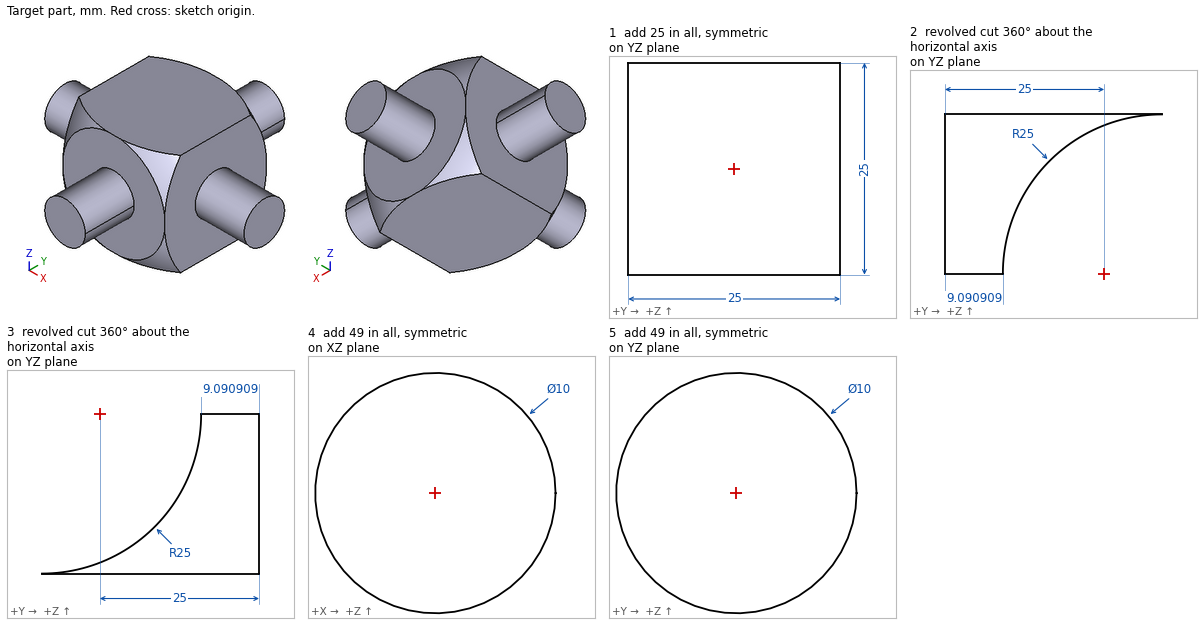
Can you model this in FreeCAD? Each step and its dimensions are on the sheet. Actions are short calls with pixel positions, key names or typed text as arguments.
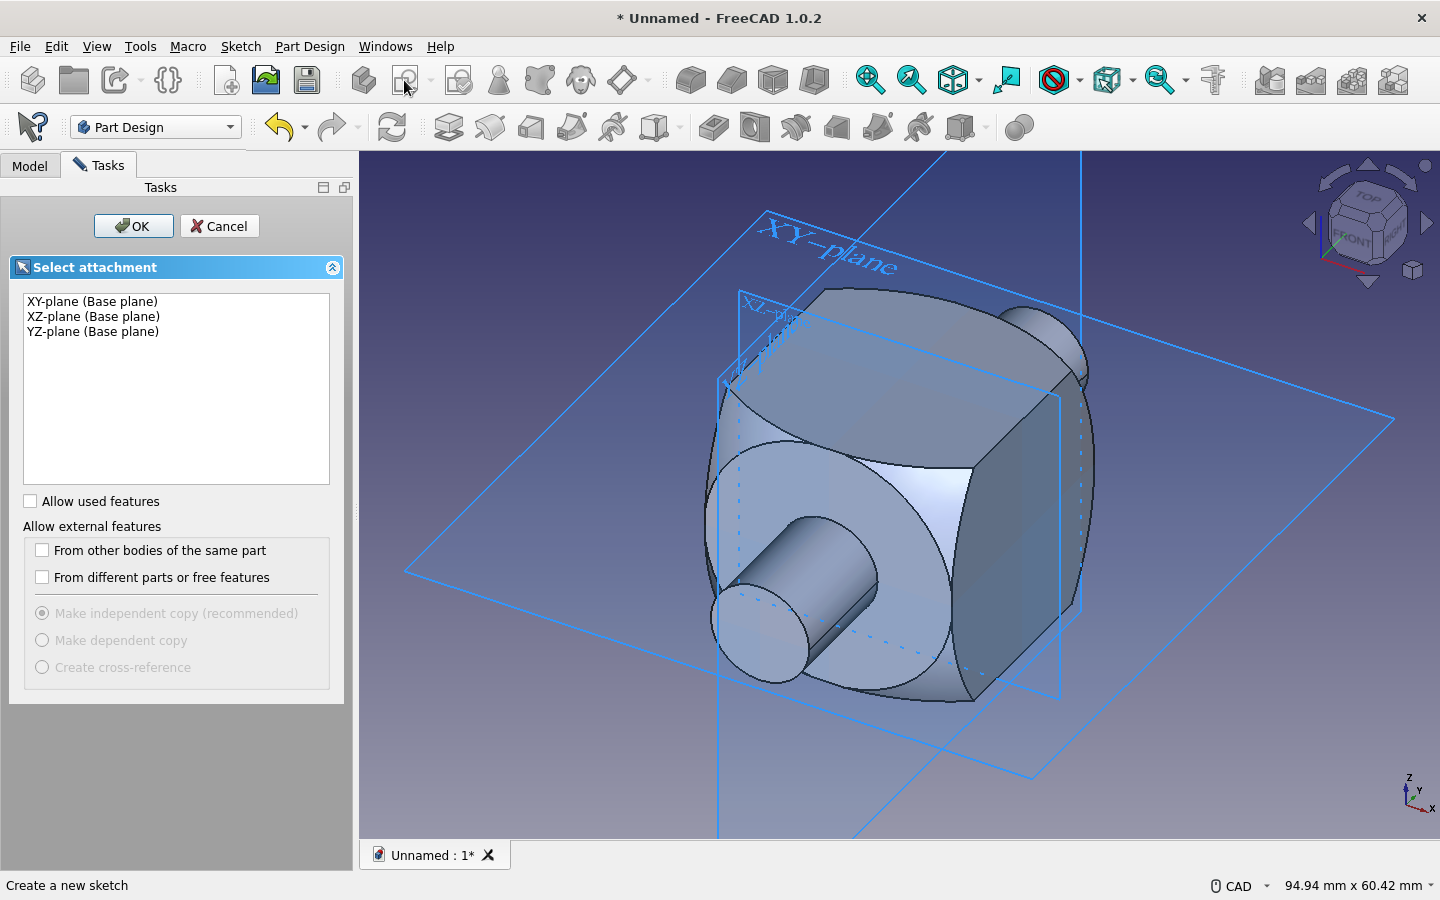
click(84, 332)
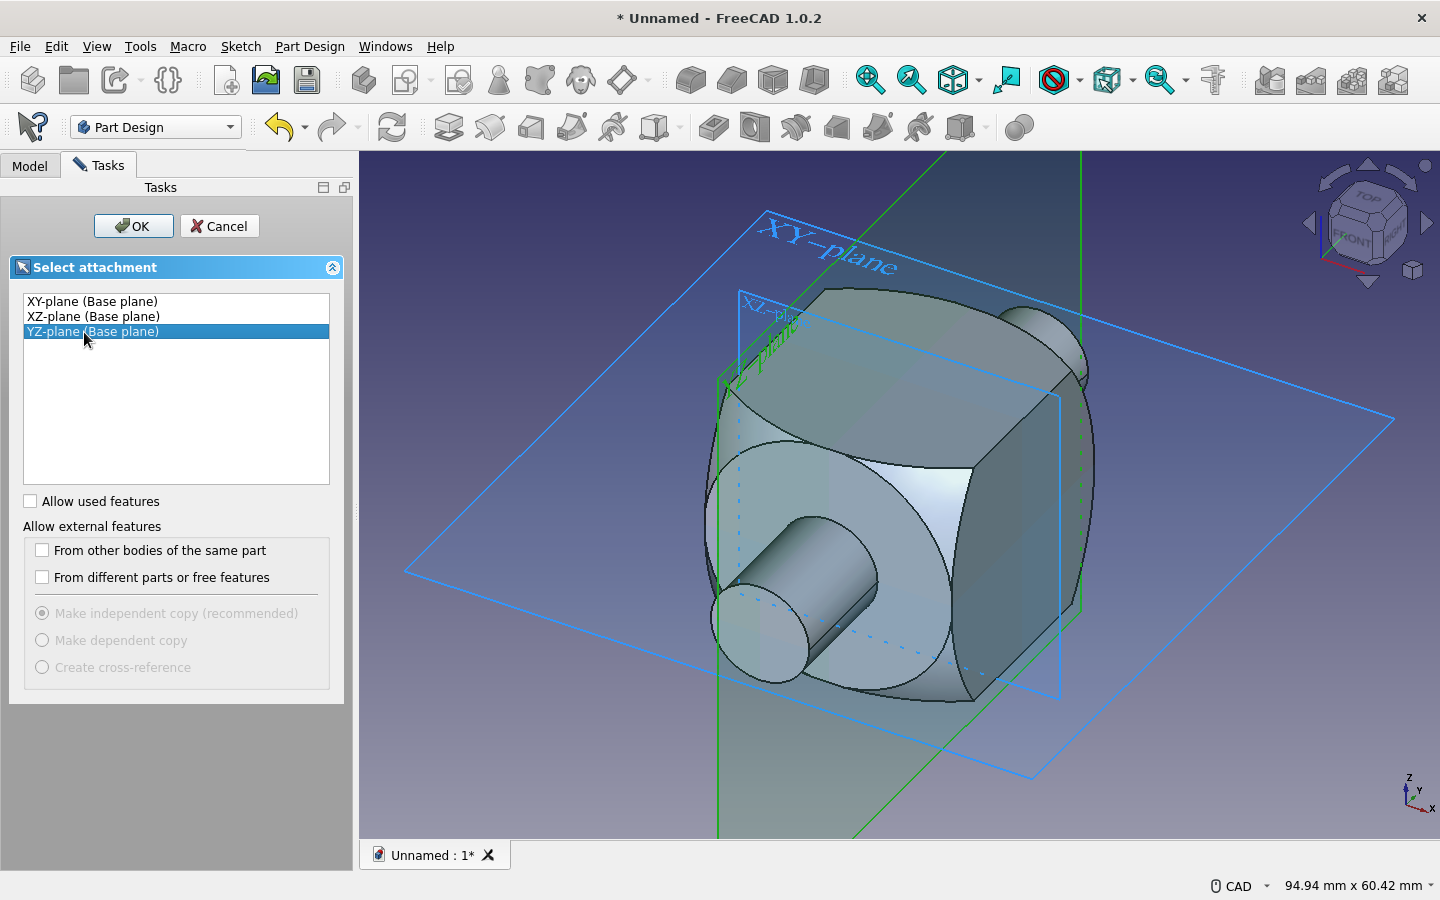
click(134, 226)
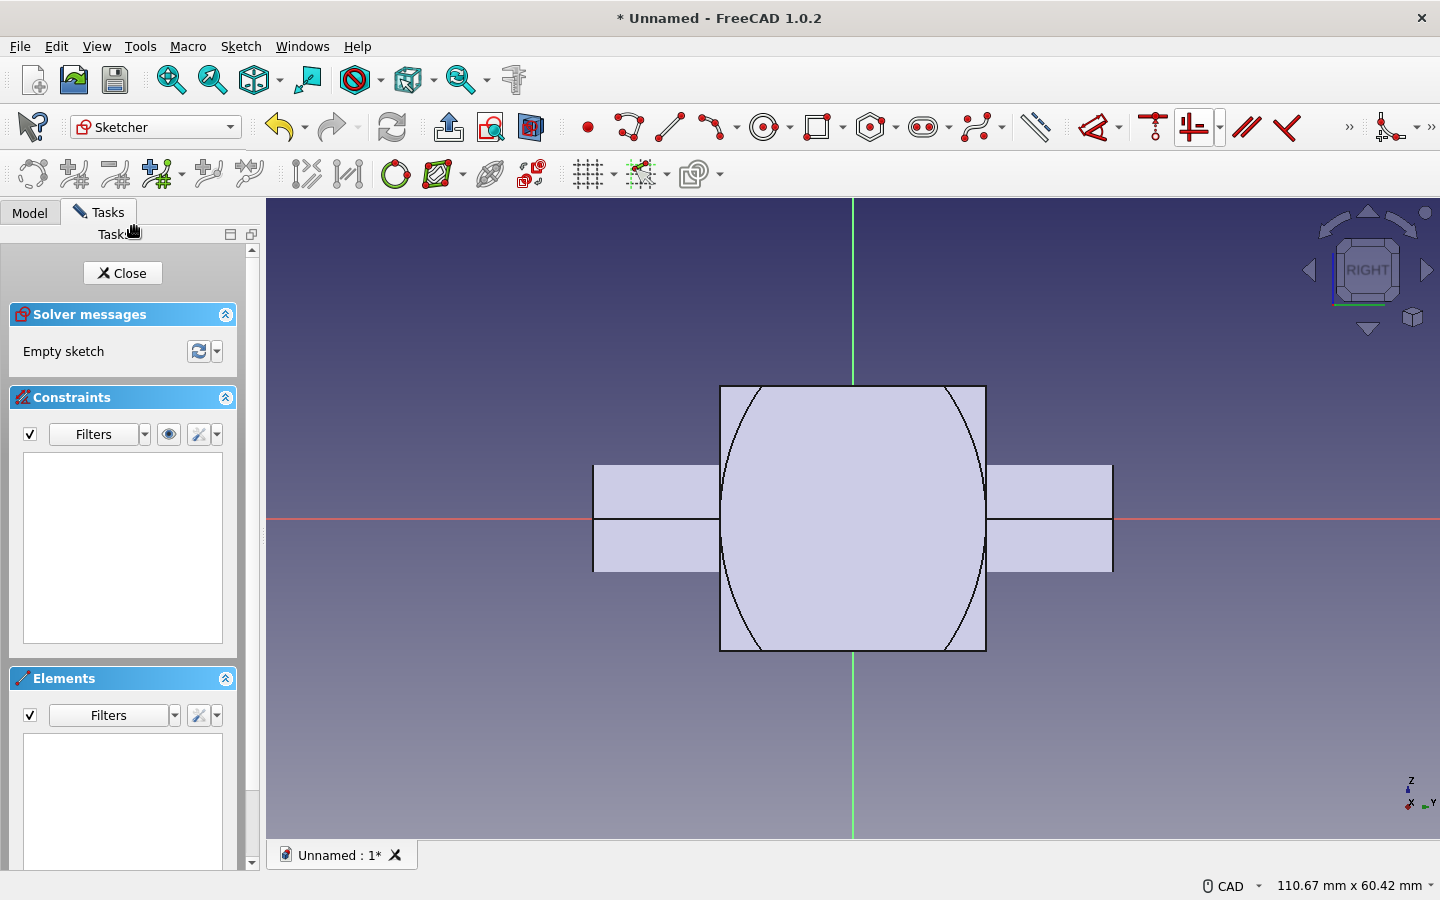
click(531, 128)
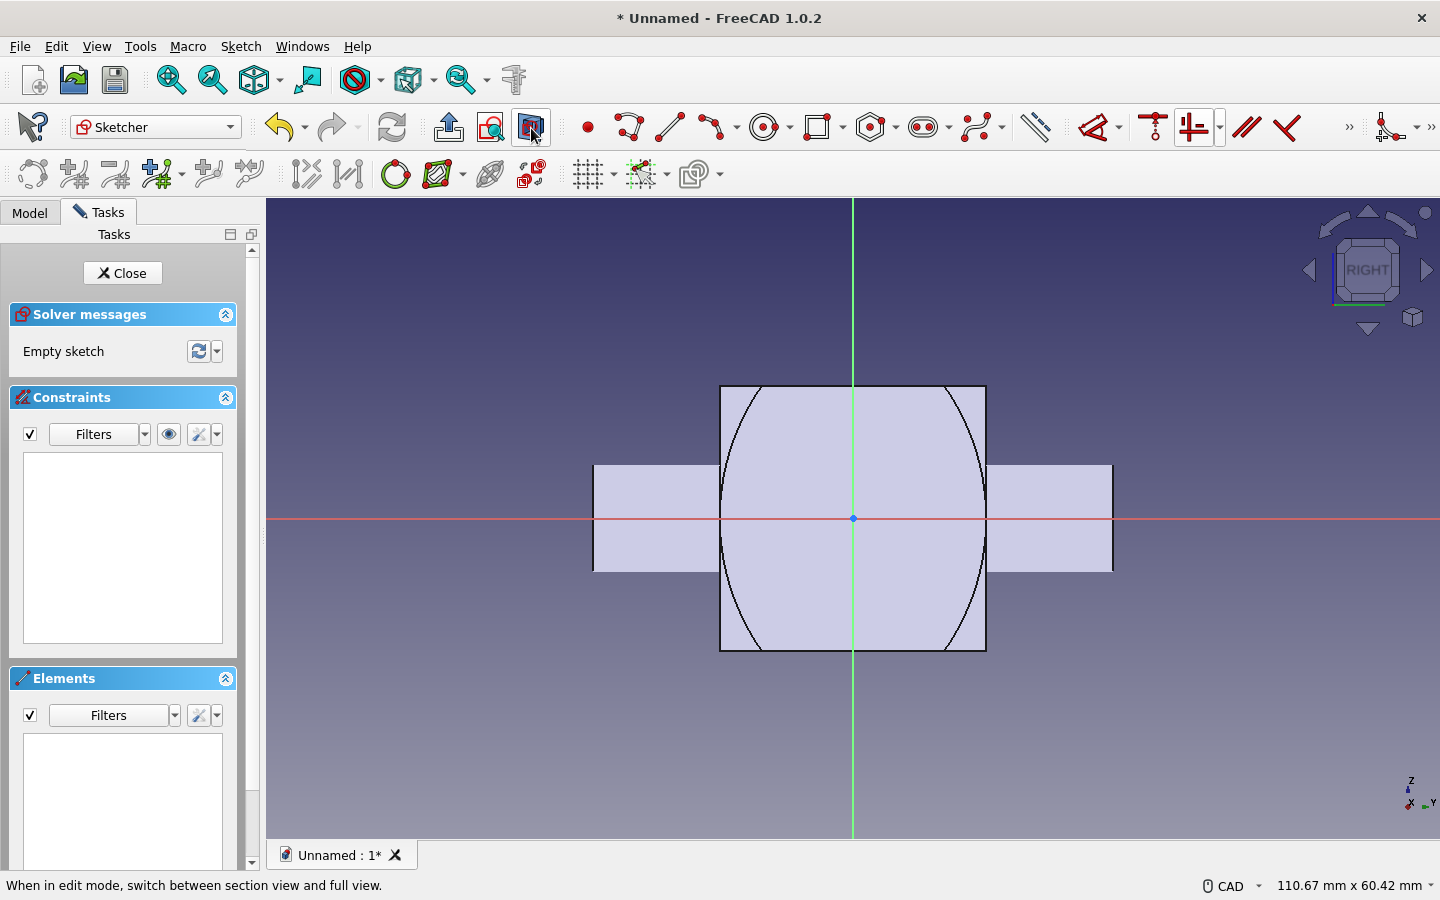
scroll(875, 518, up, 7)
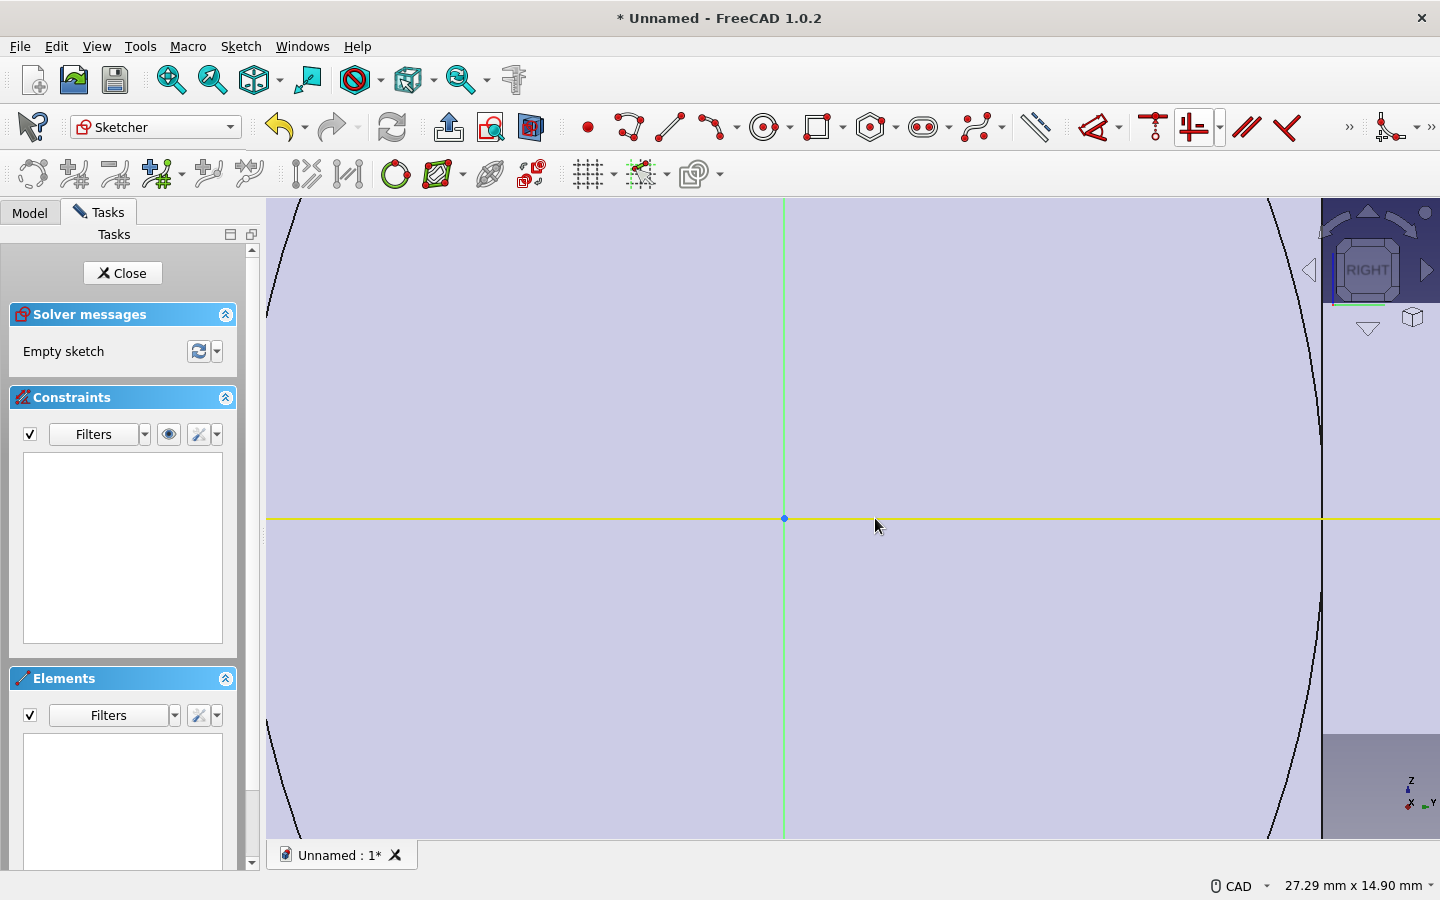
key(g)
key(c)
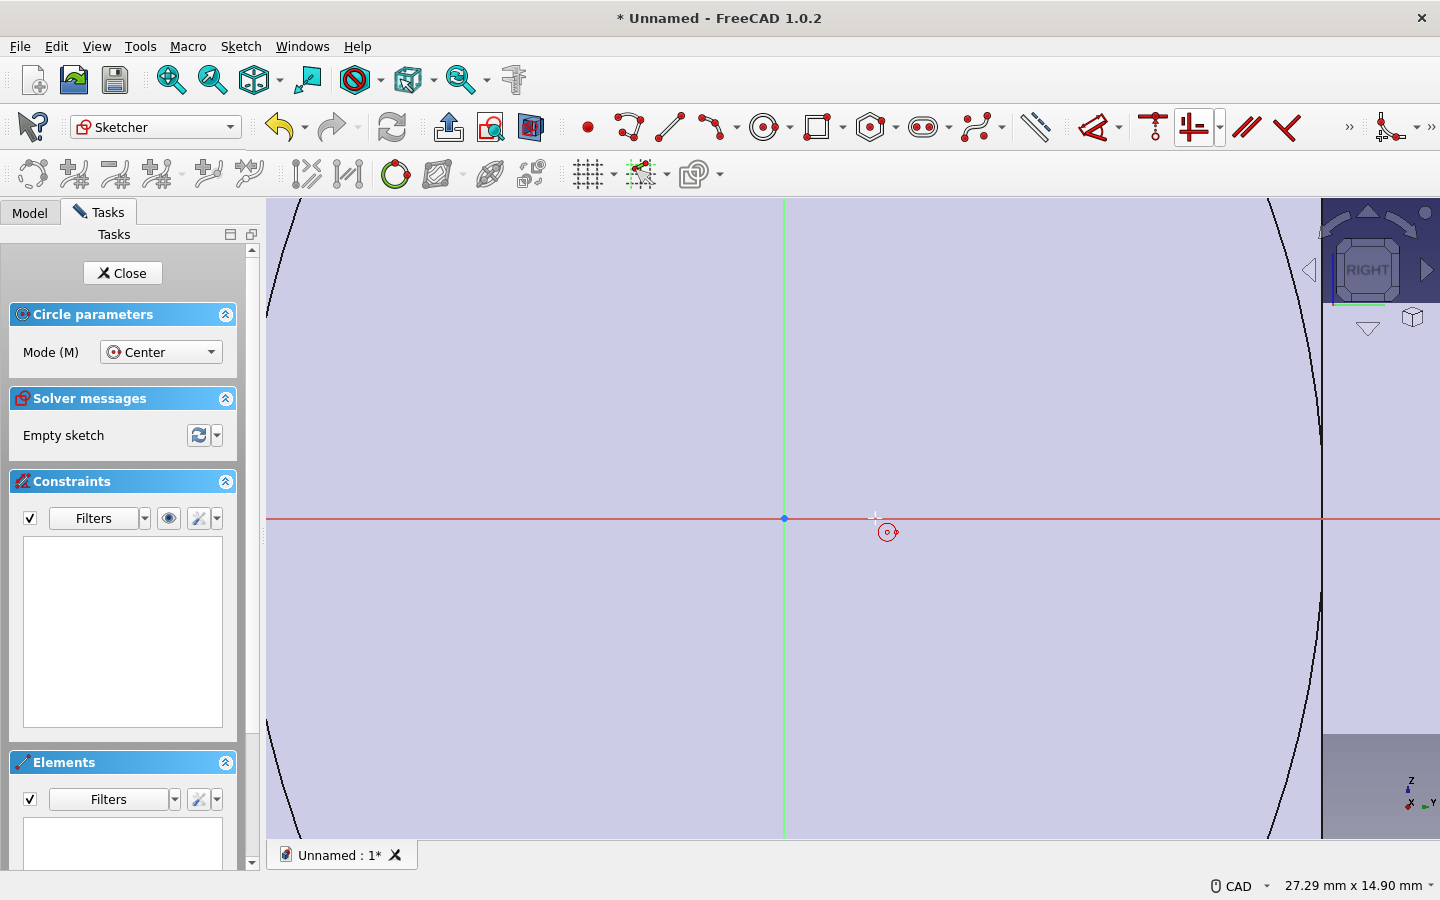
click(784, 518)
click(936, 366)
key(Escape)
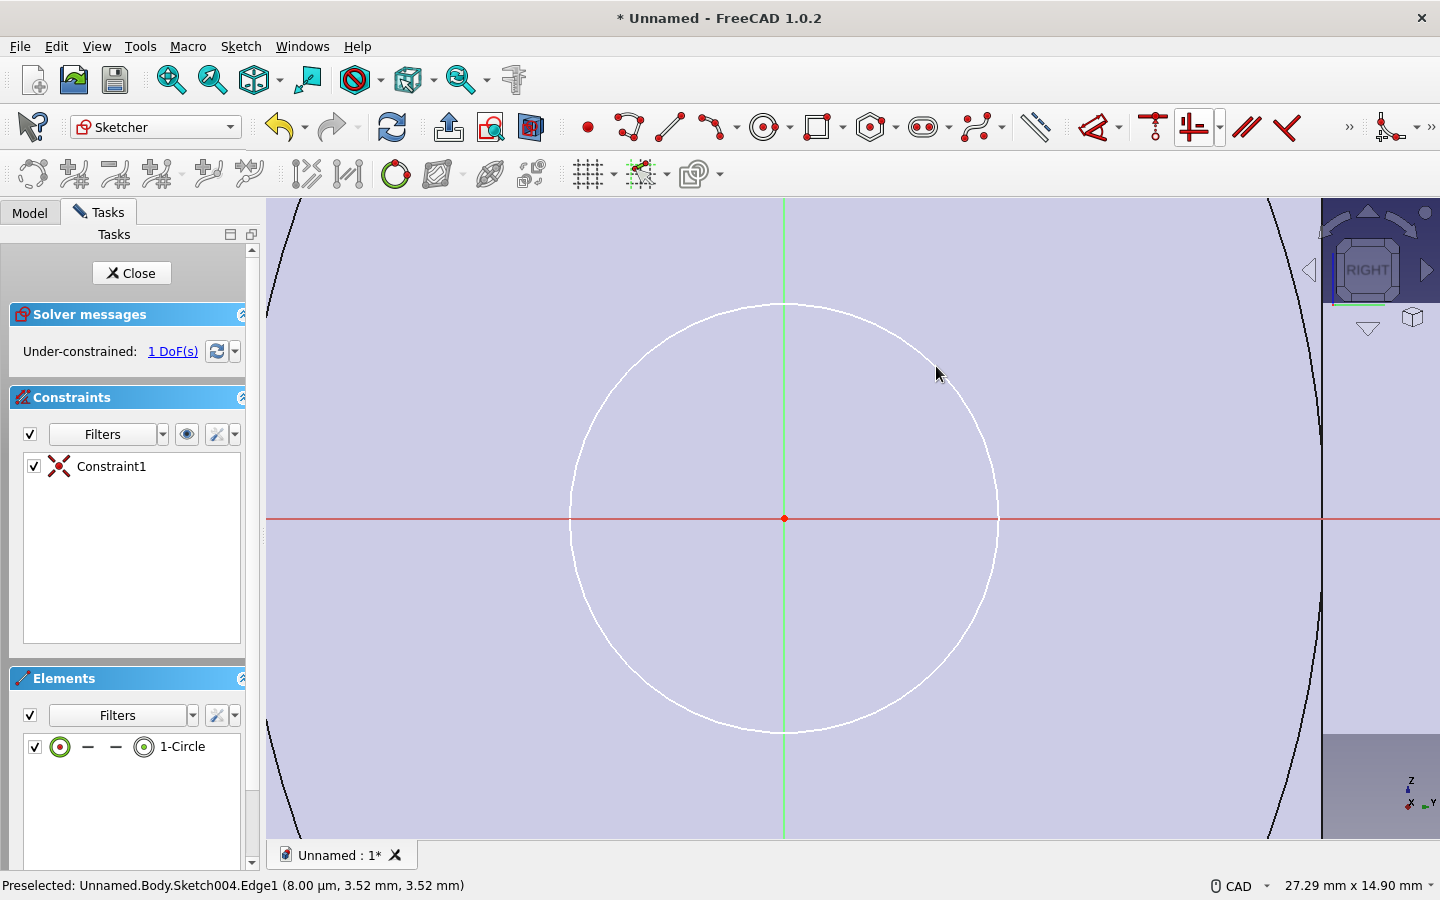
click(1092, 128)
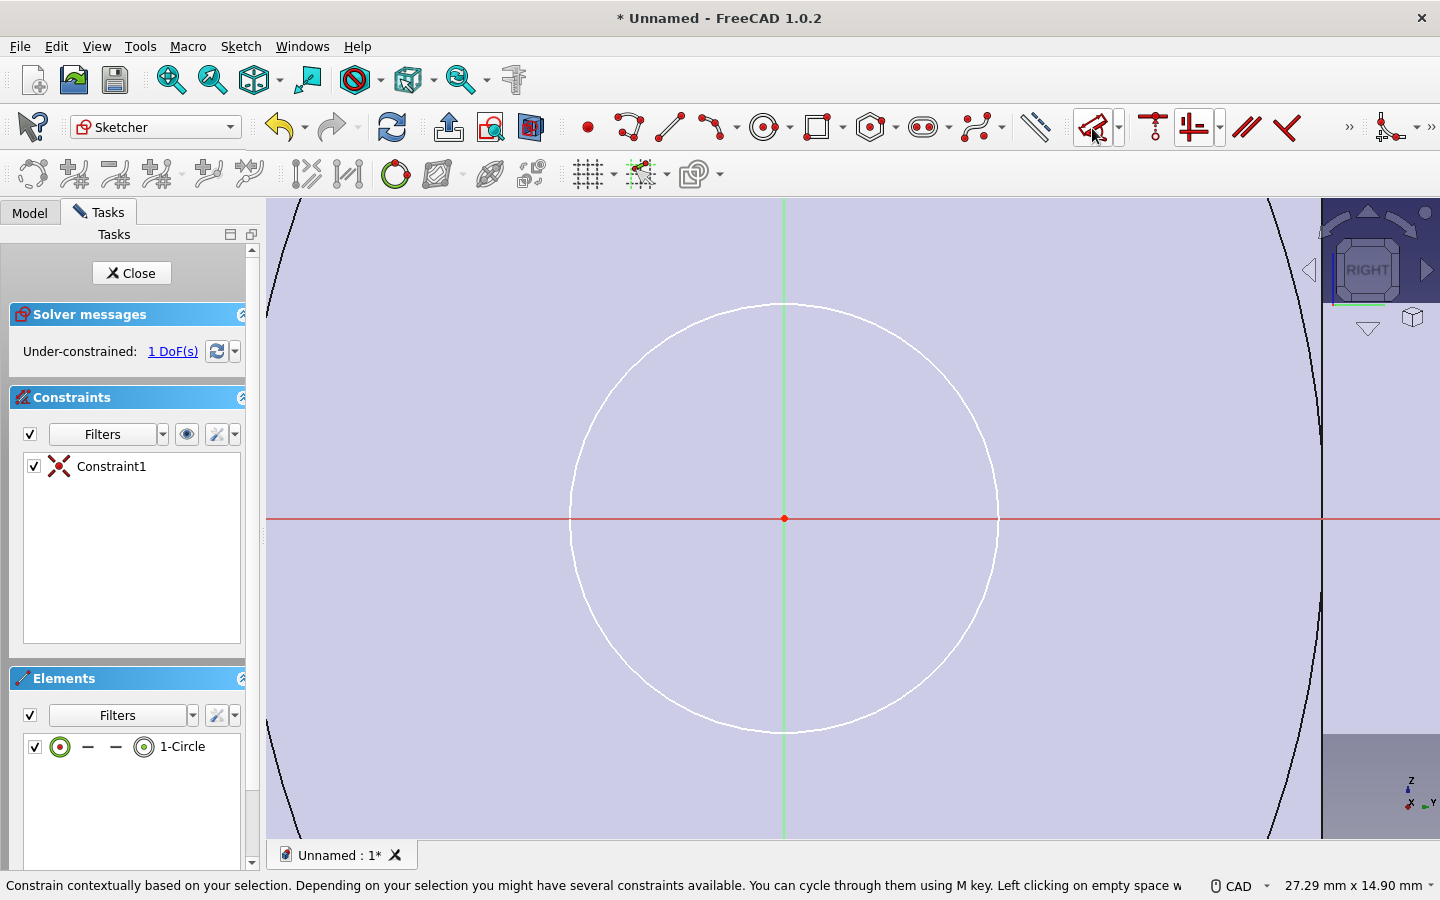
click(935, 366)
click(958, 343)